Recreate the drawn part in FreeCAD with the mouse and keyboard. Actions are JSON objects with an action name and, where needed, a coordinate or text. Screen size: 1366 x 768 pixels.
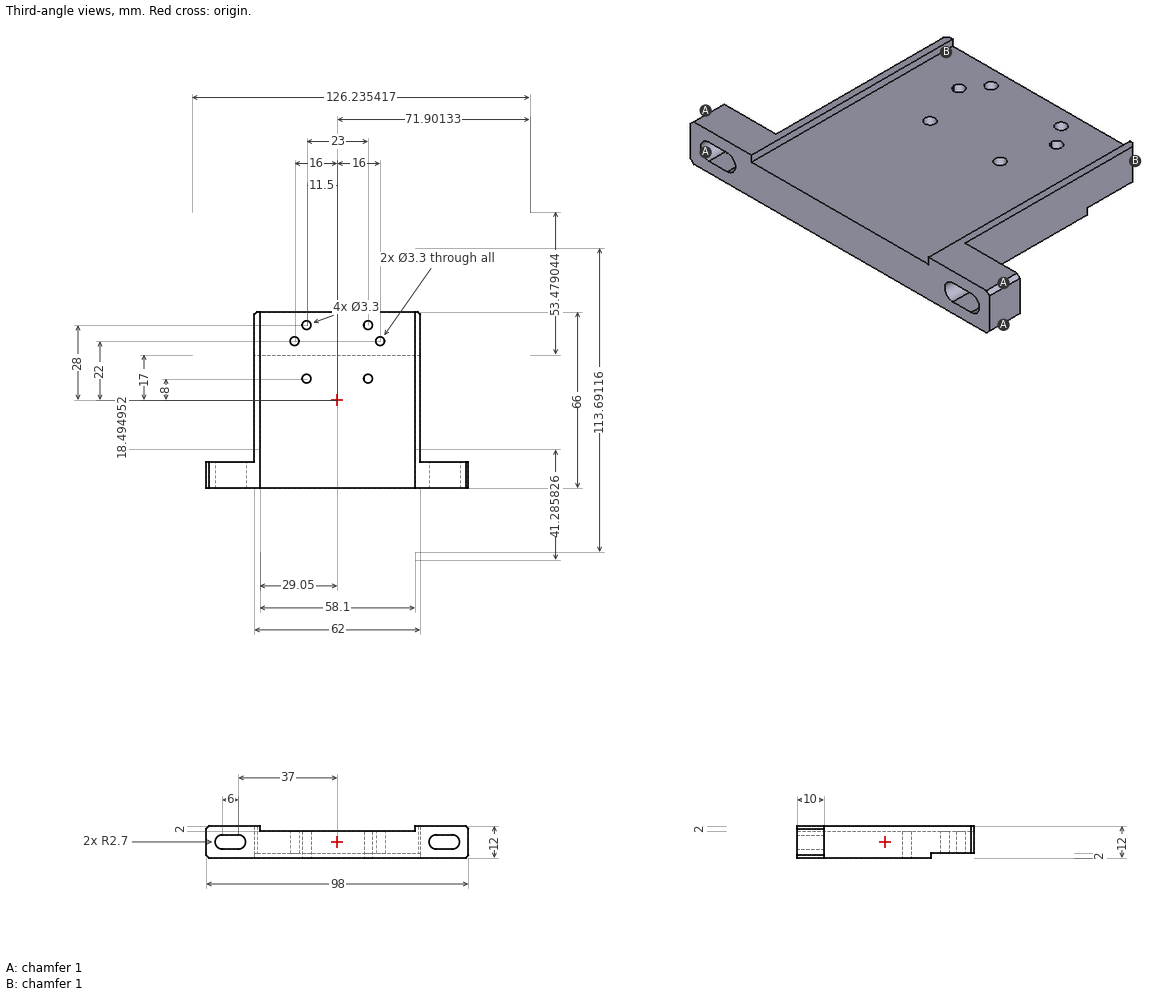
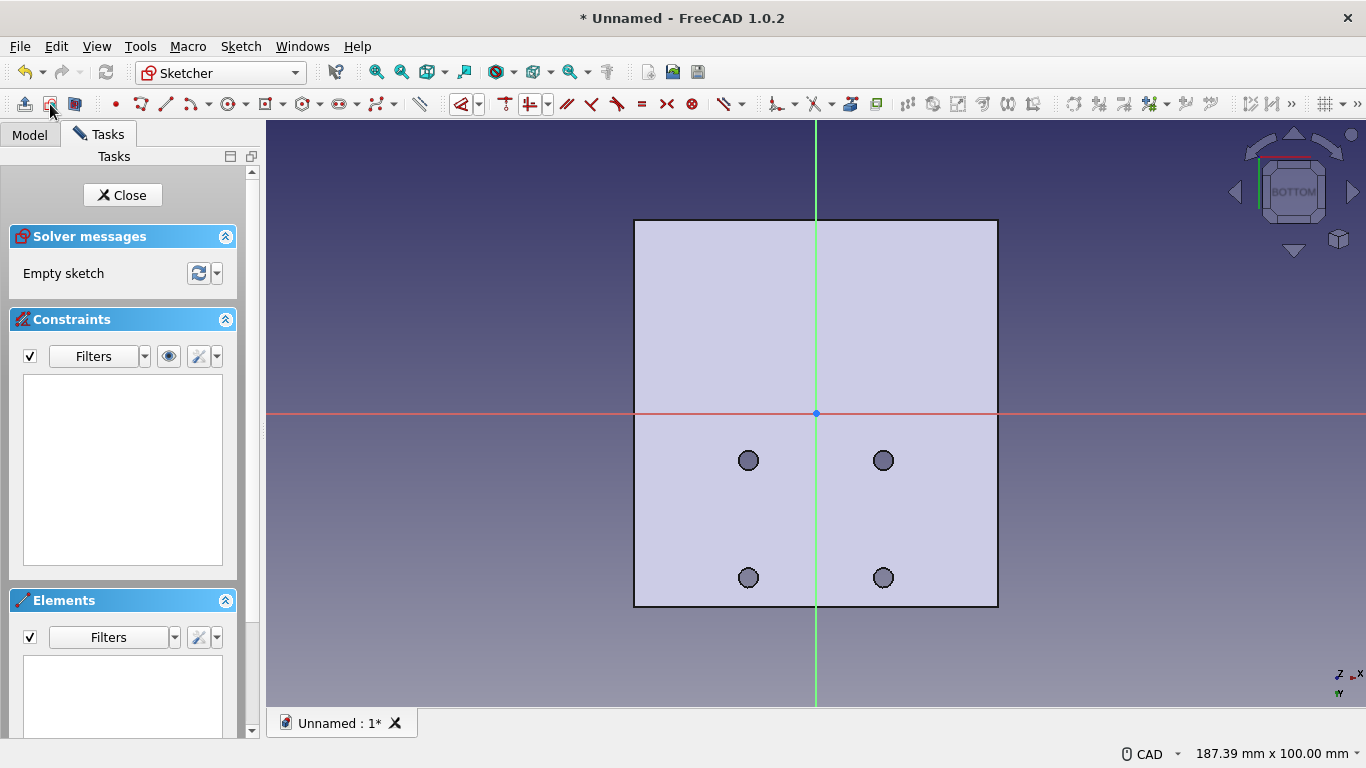
{"action": "scroll", "coordinate": [856, 523], "scroll_direction": "up", "scroll_amount": 5}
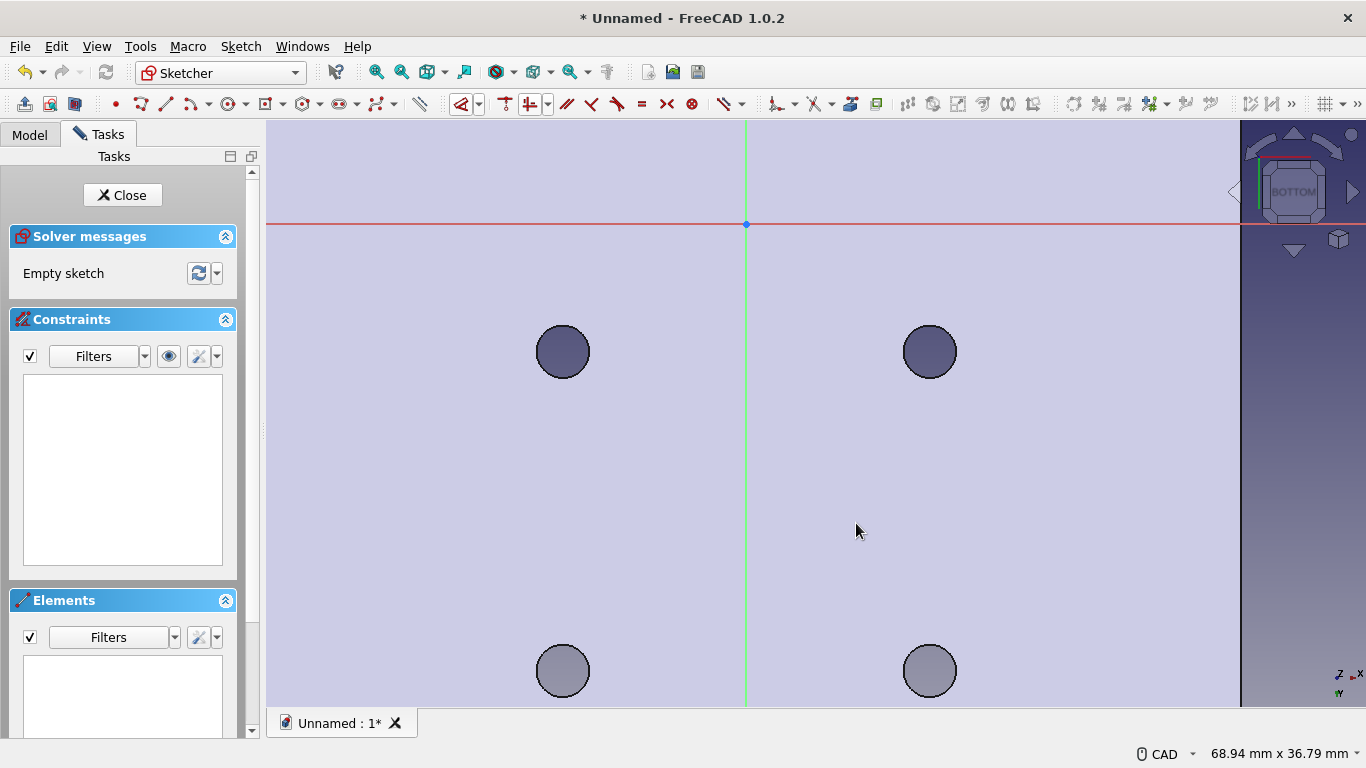
{"action": "left_click", "coordinate": [228, 104]}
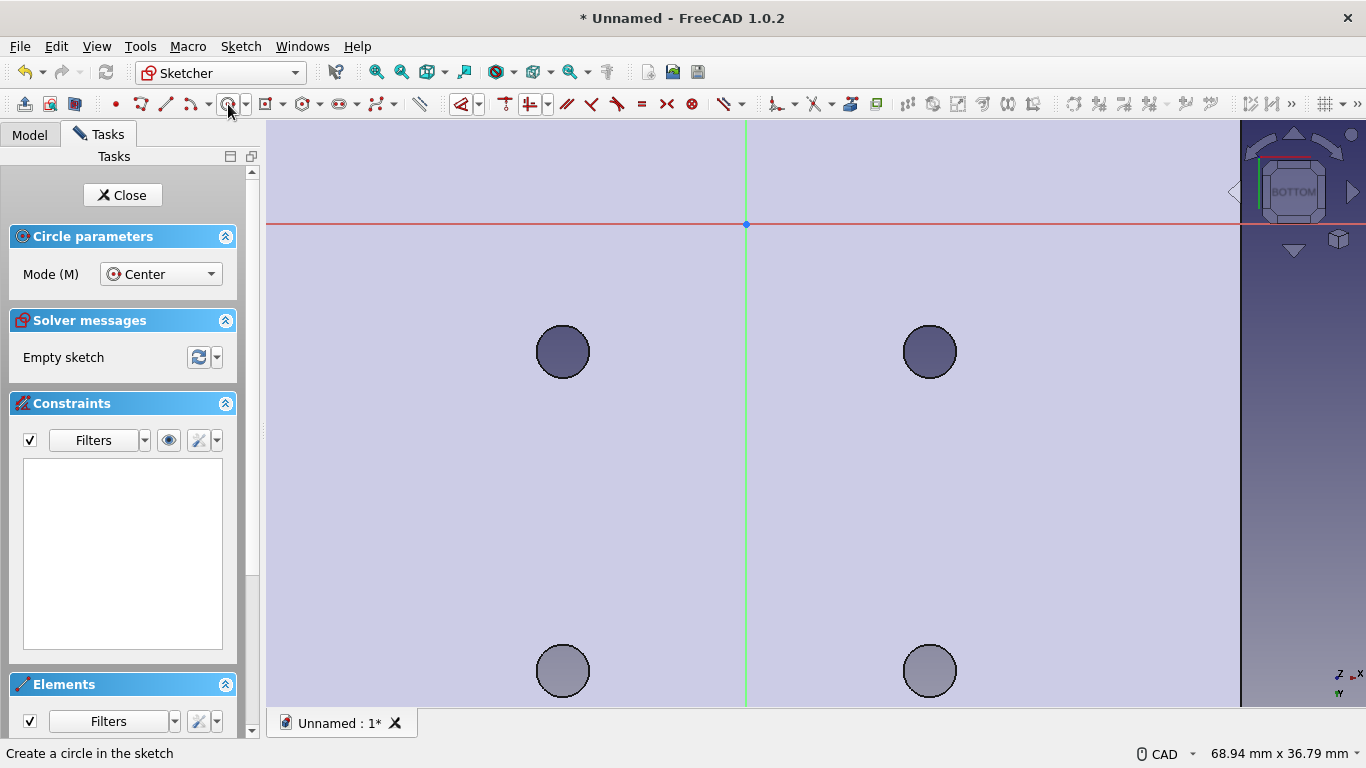
{"action": "left_click", "coordinate": [1002, 575]}
{"action": "mouse_move", "coordinate": [1020, 557]}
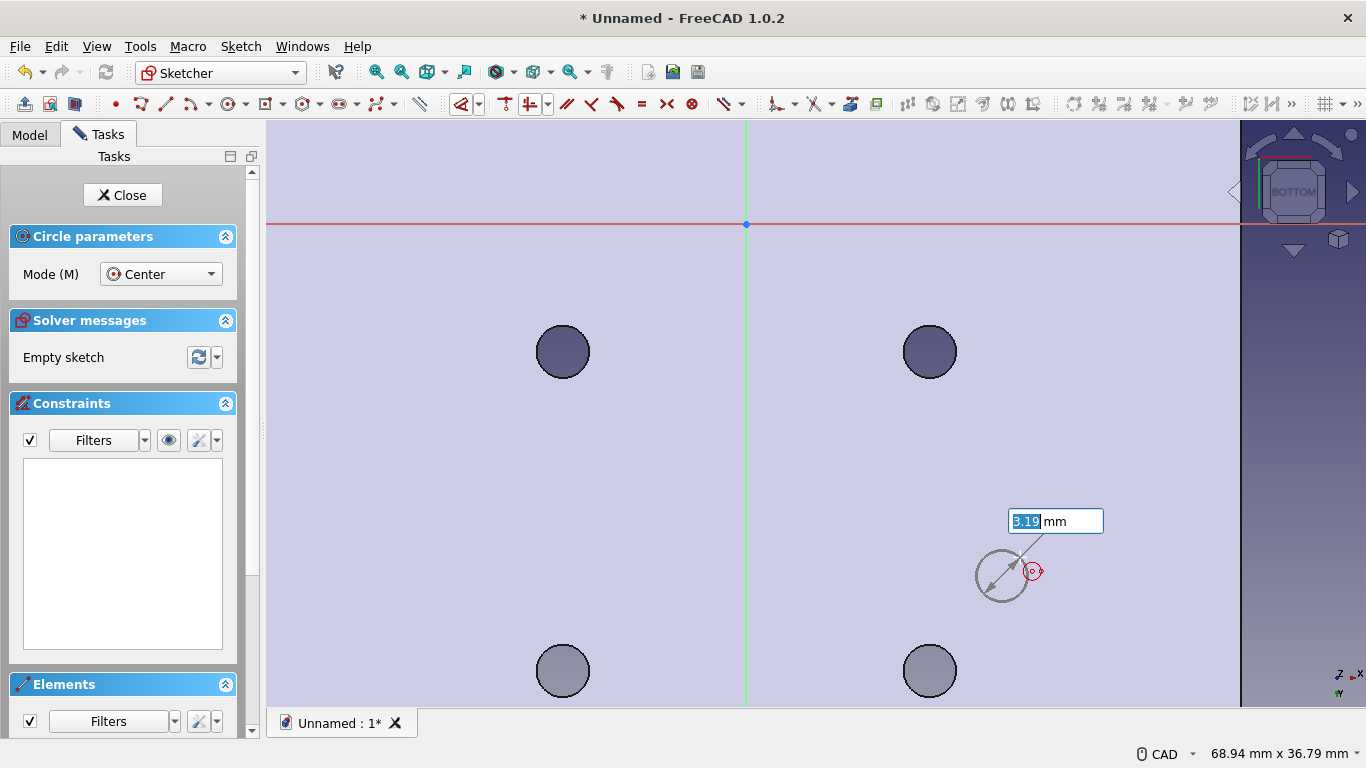
{"action": "type", "text": "3.3"}
{"action": "key", "text": "Return"}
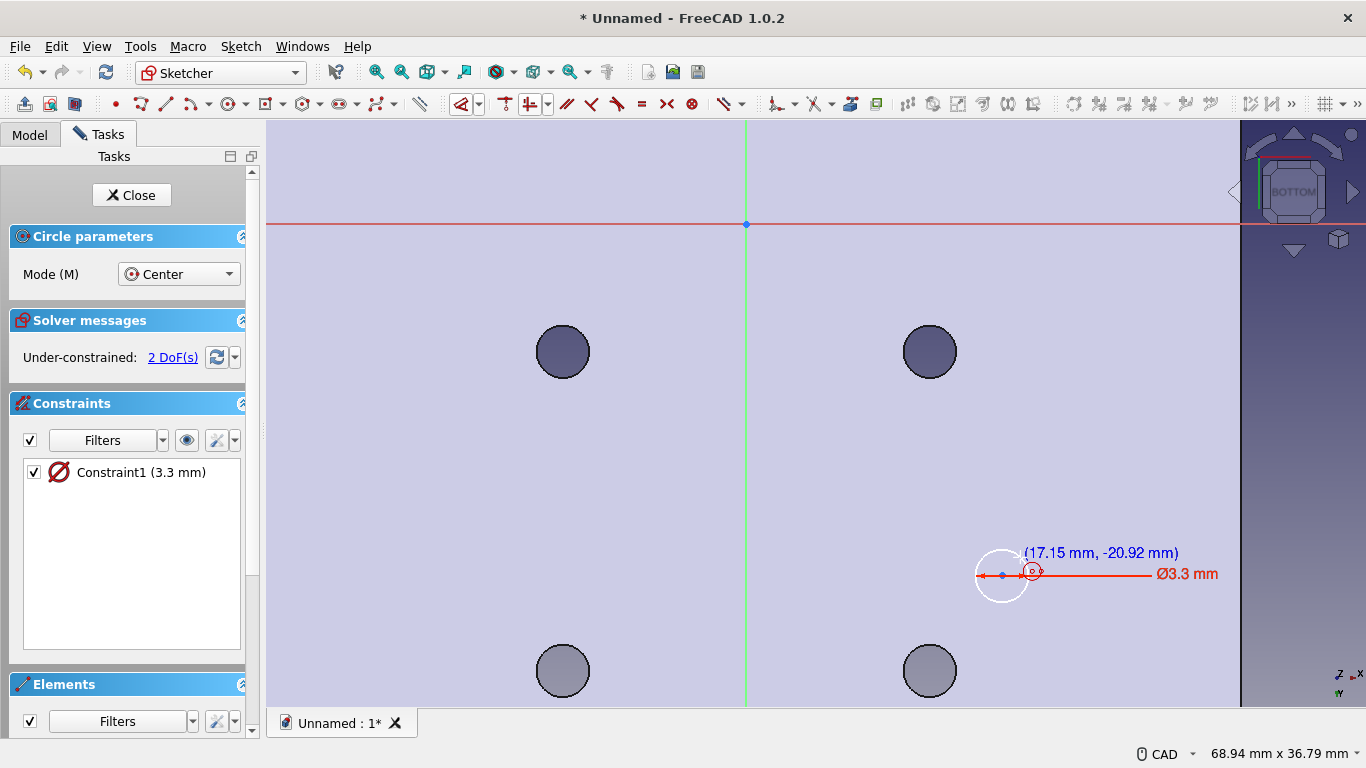
{"action": "left_click", "coordinate": [491, 575]}
{"action": "mouse_move", "coordinate": [510, 557]}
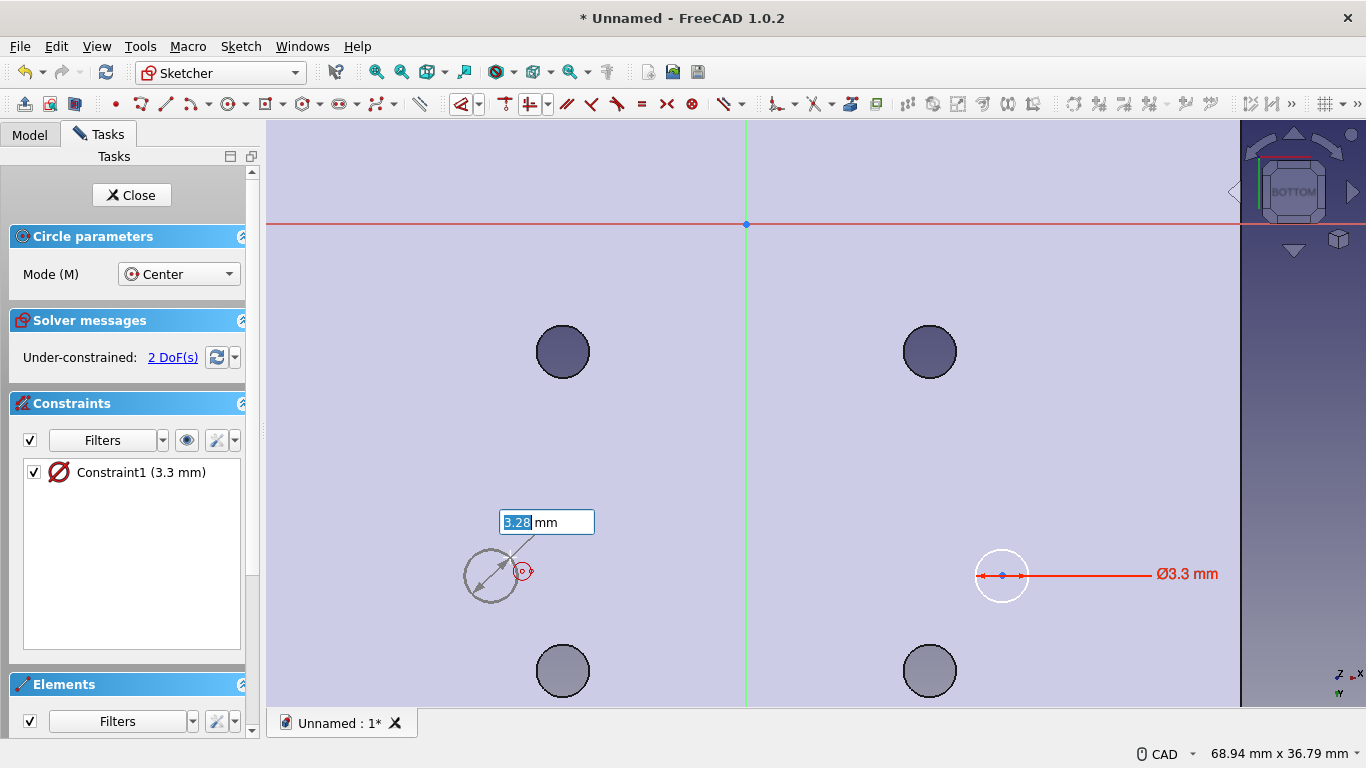
{"action": "type", "text": "3.3"}
{"action": "key", "text": "Return"}
{"action": "key", "text": "Escape"}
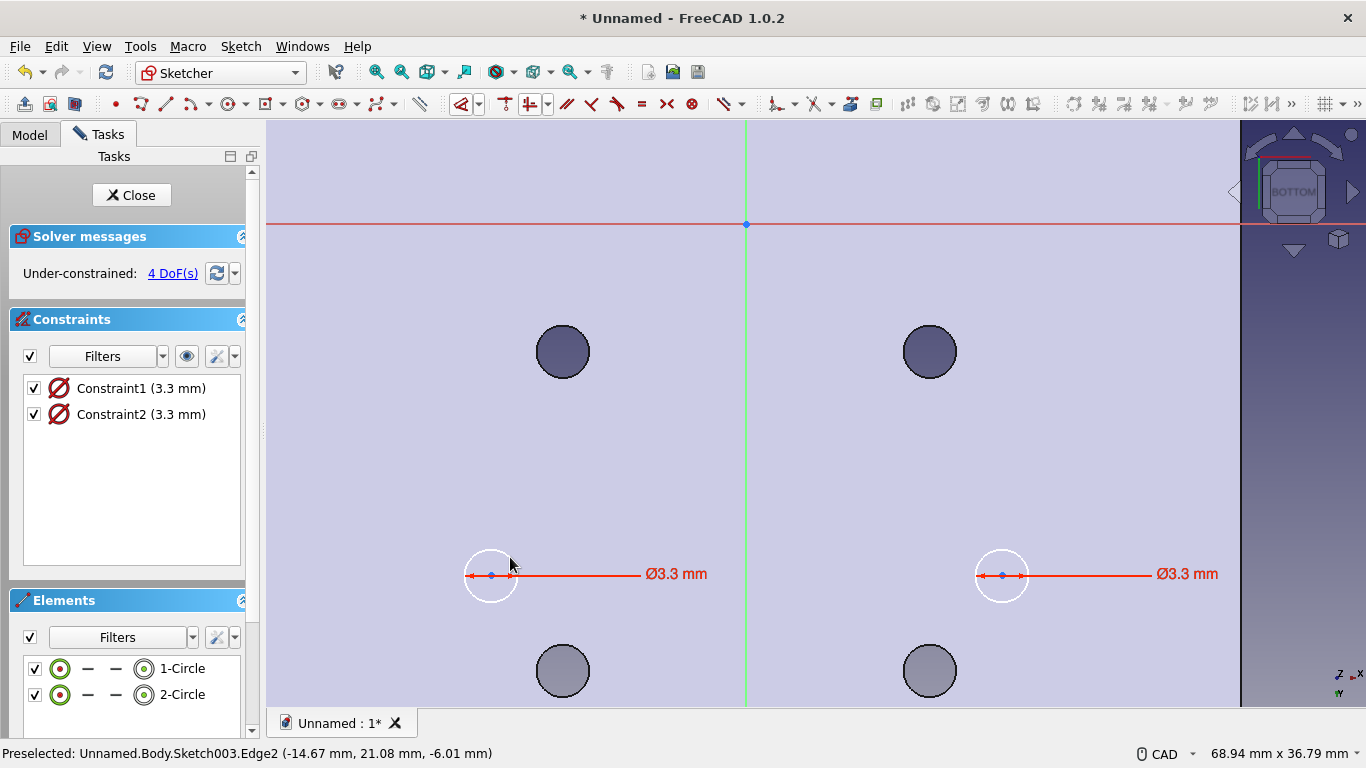
{"action": "left_click", "coordinate": [1002, 576]}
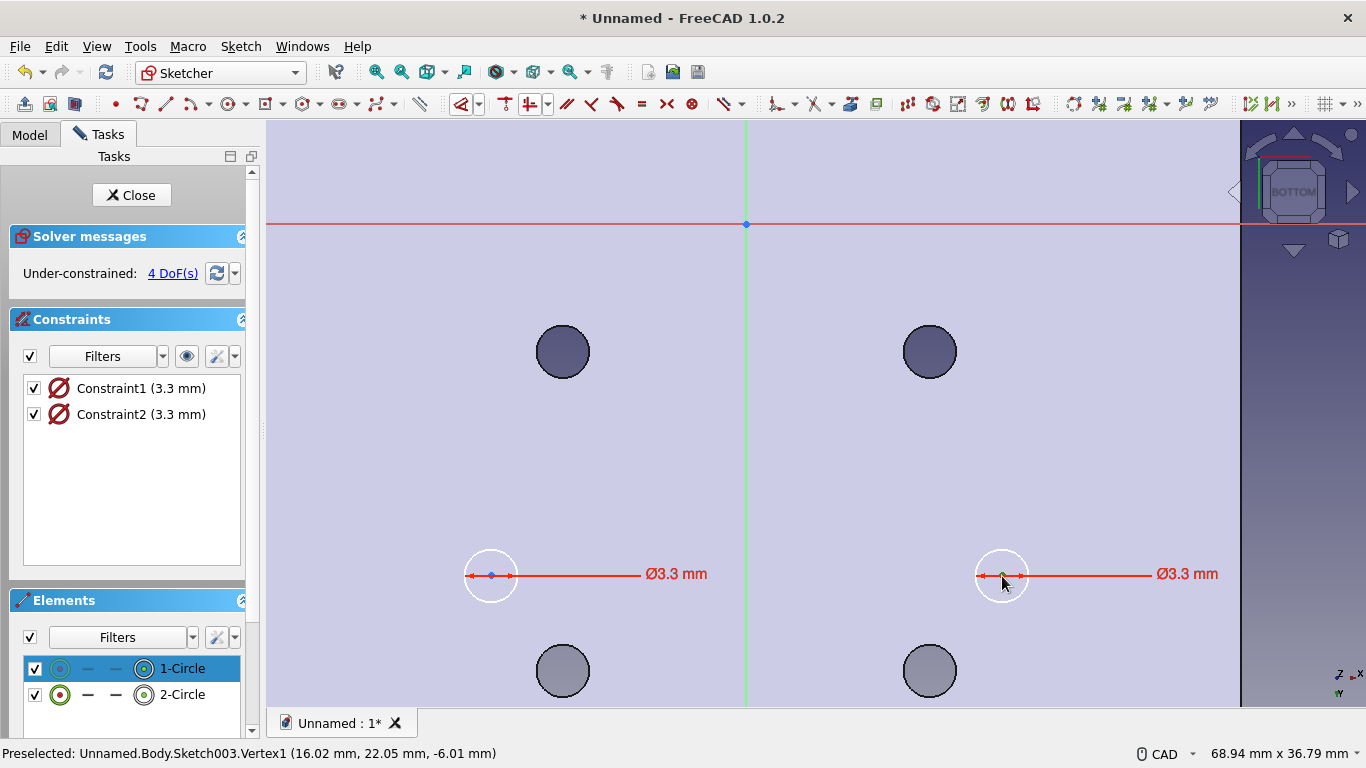
{"action": "left_click", "coordinate": [491, 576]}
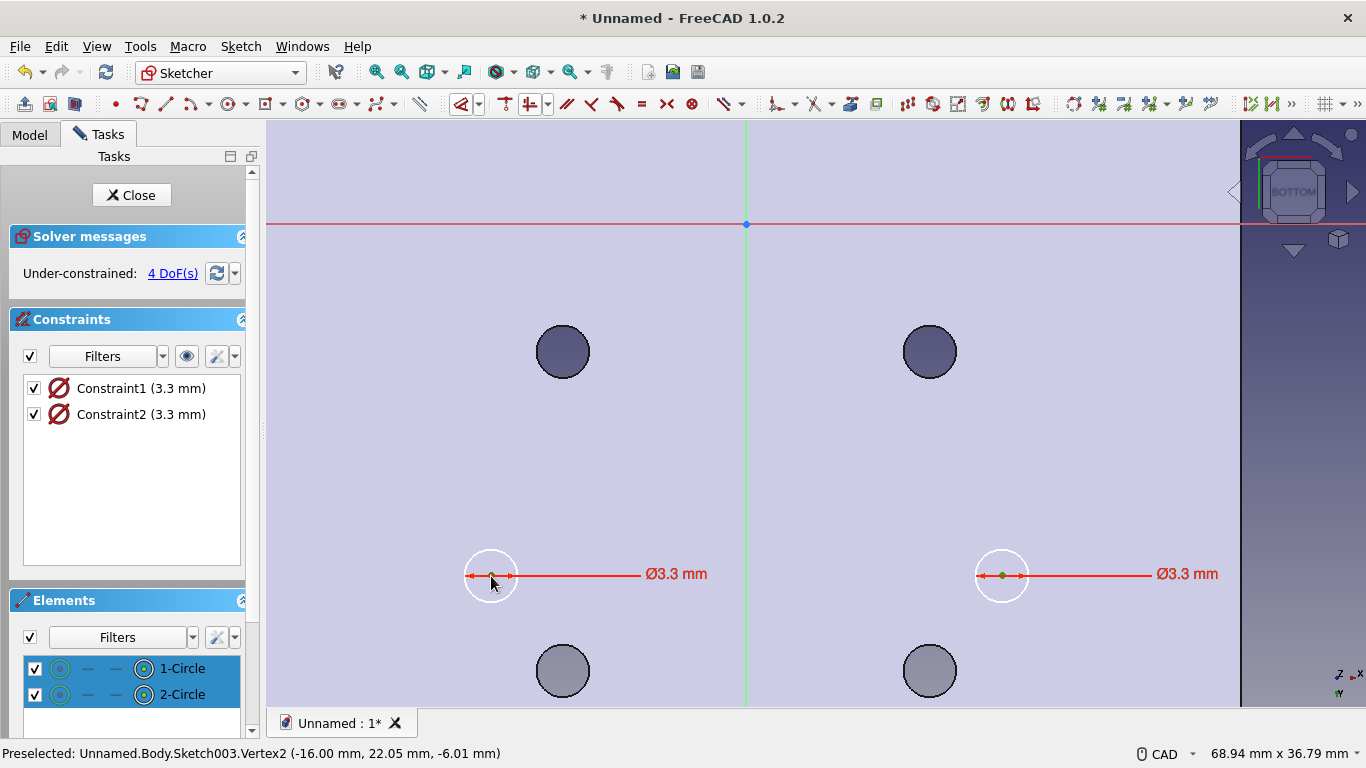
{"action": "key", "text": "h"}